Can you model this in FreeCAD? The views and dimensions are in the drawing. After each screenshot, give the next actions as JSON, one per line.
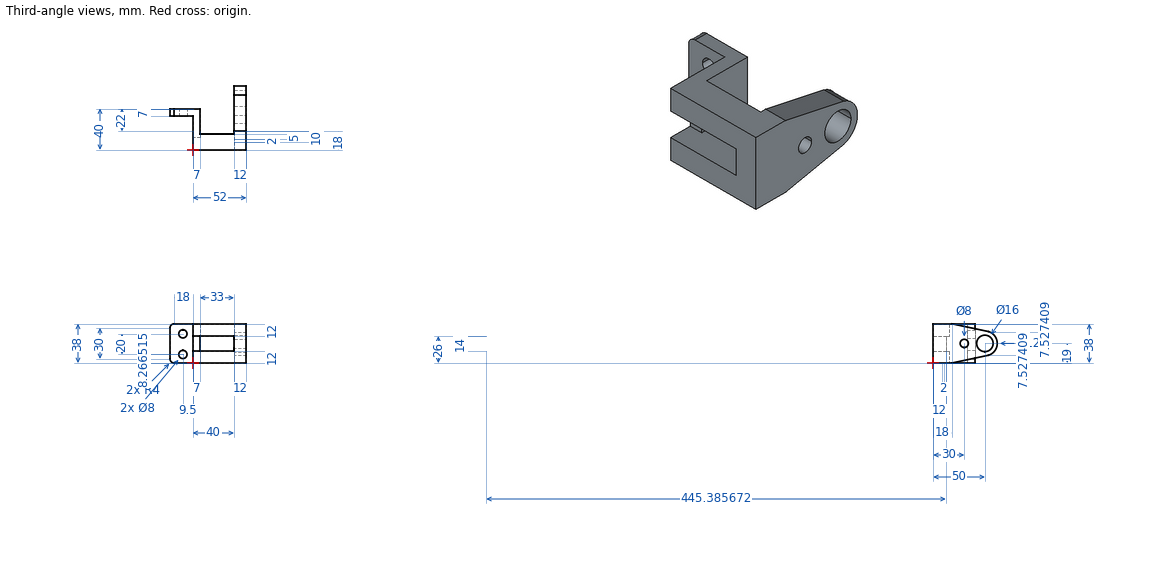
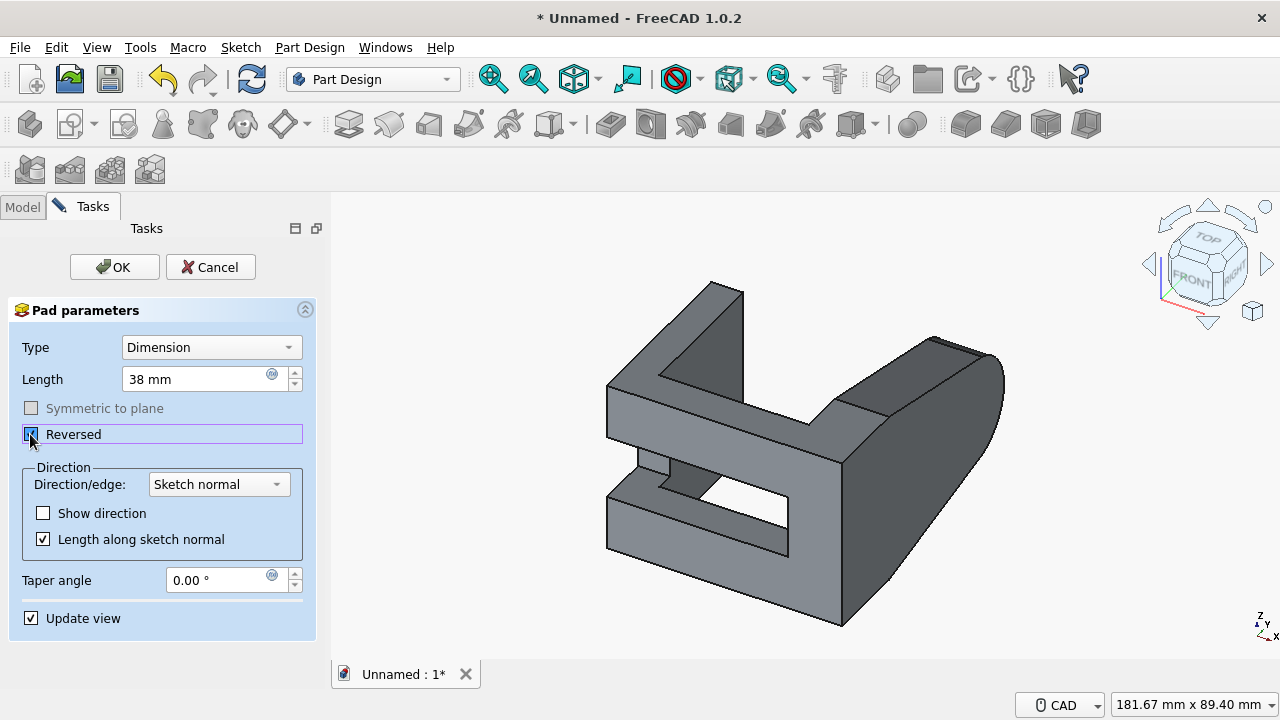
{"action": "left_click", "coordinate": [115, 267]}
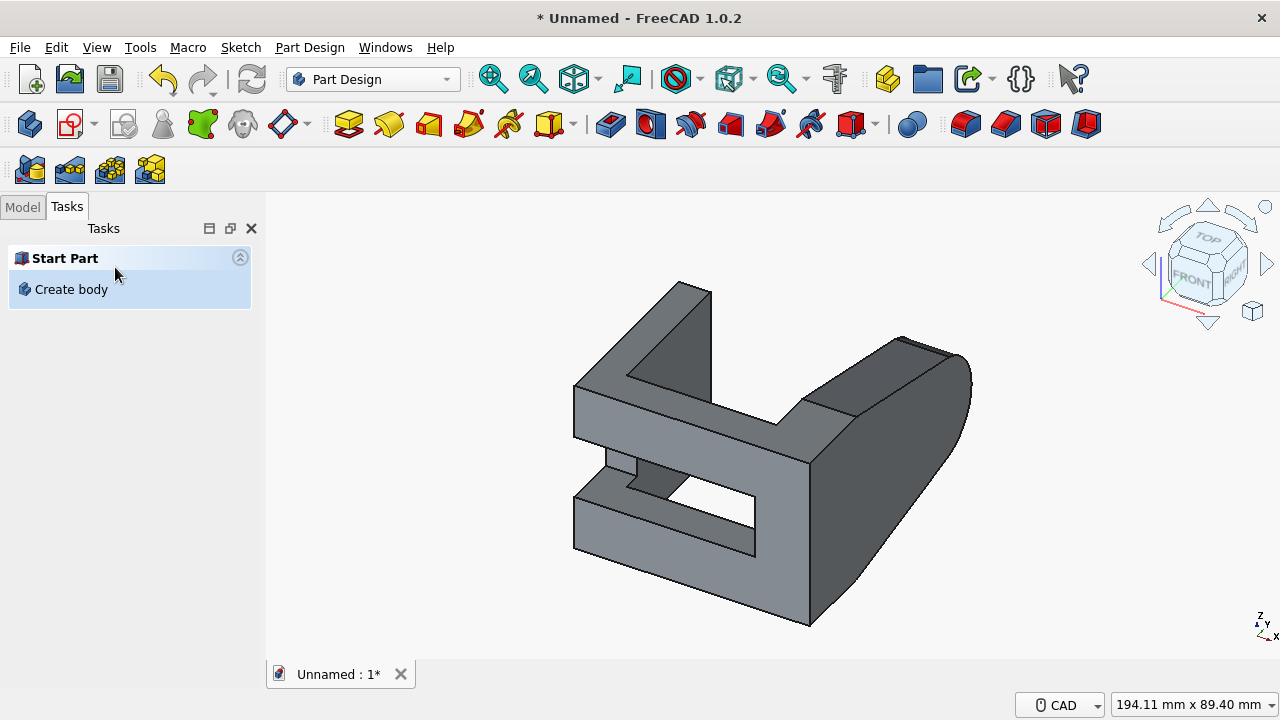
{"action": "key", "text": "4"}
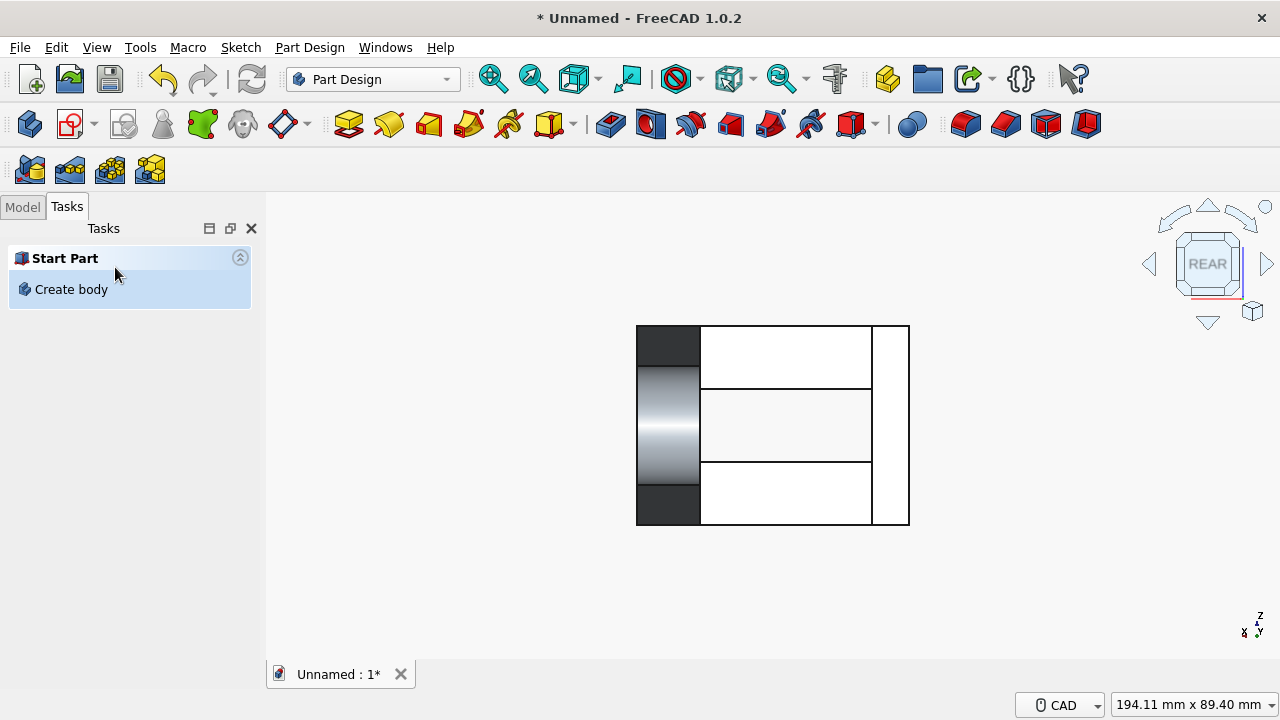
{"action": "left_click", "coordinate": [494, 80]}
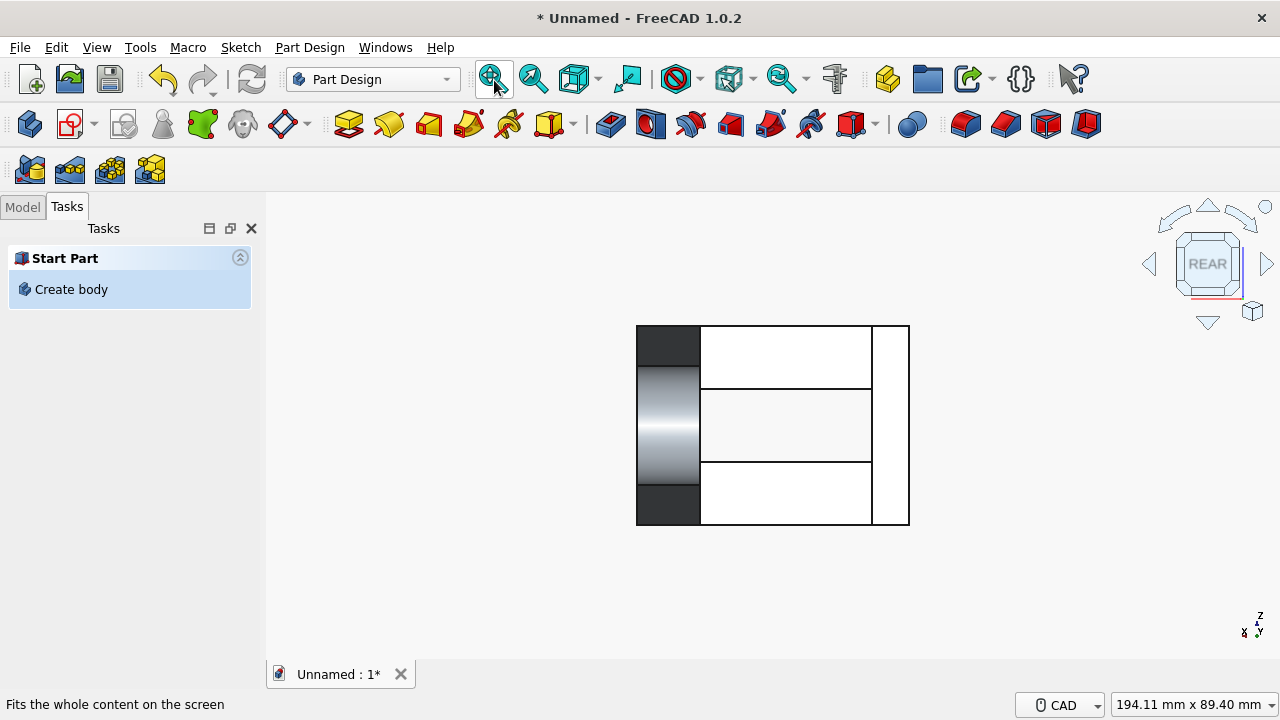
{"action": "left_click", "coordinate": [891, 368]}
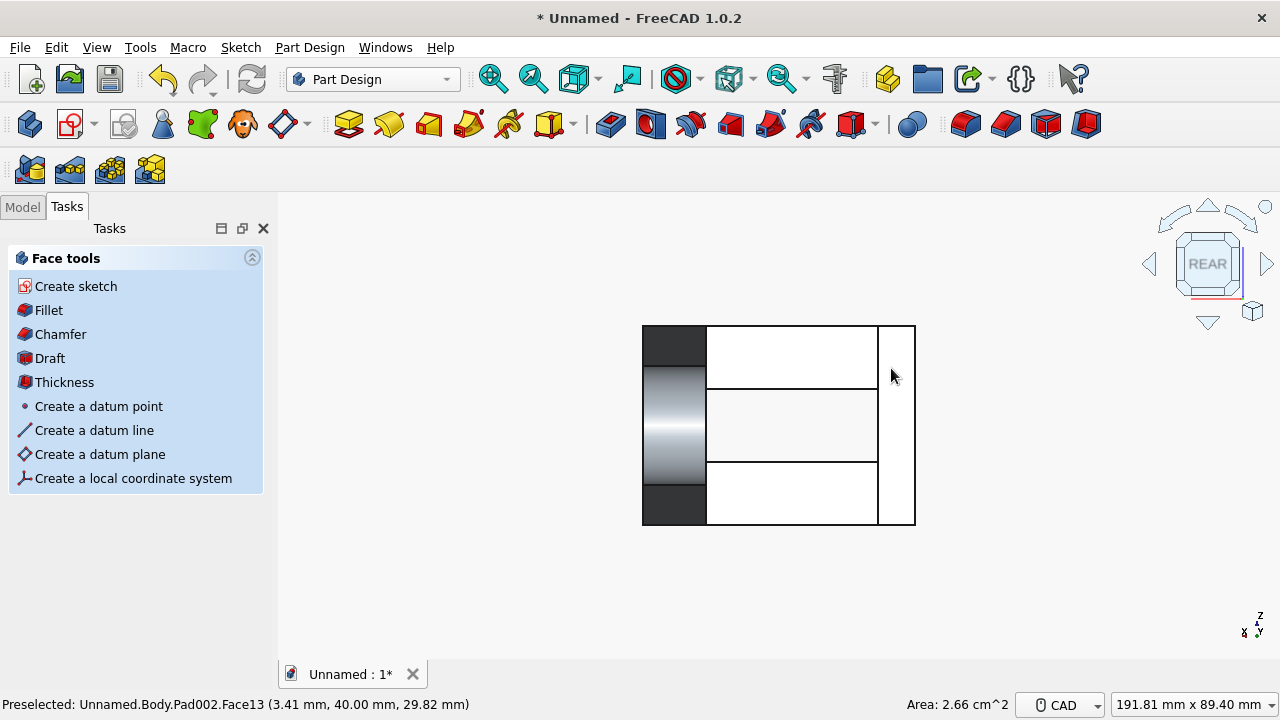
{"action": "left_click", "coordinate": [70, 124]}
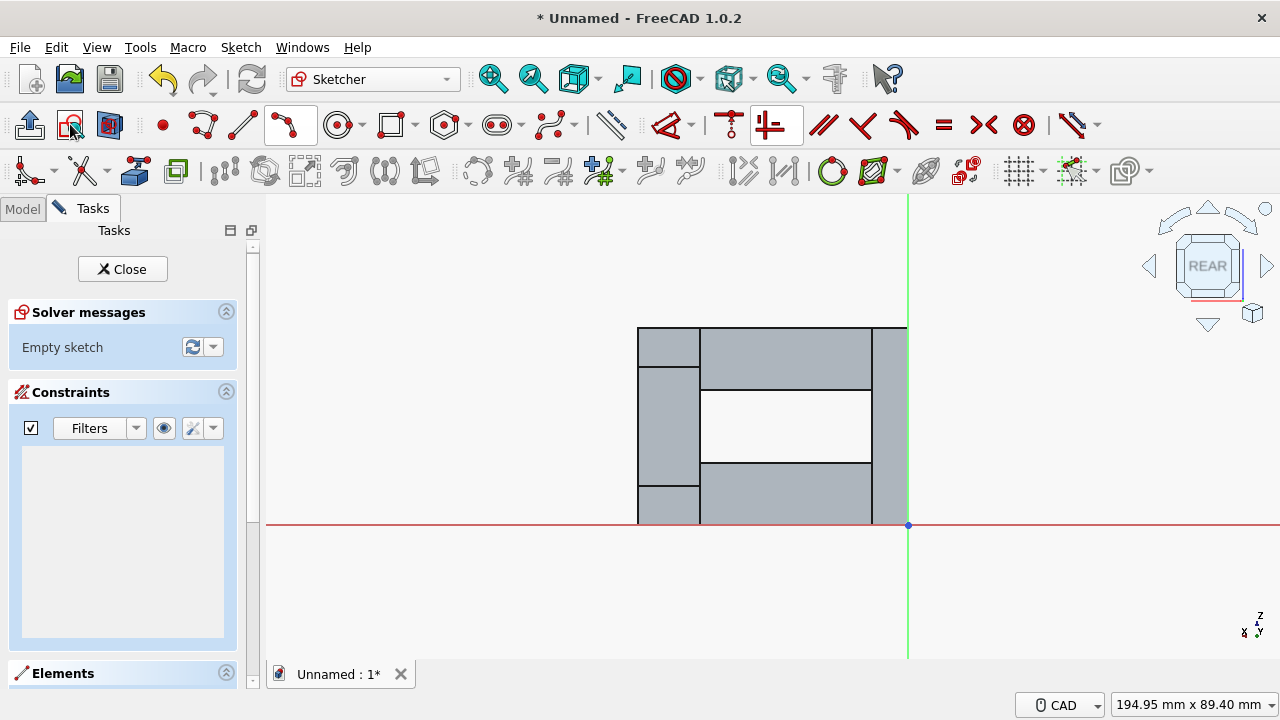
{"action": "left_click", "coordinate": [110, 126]}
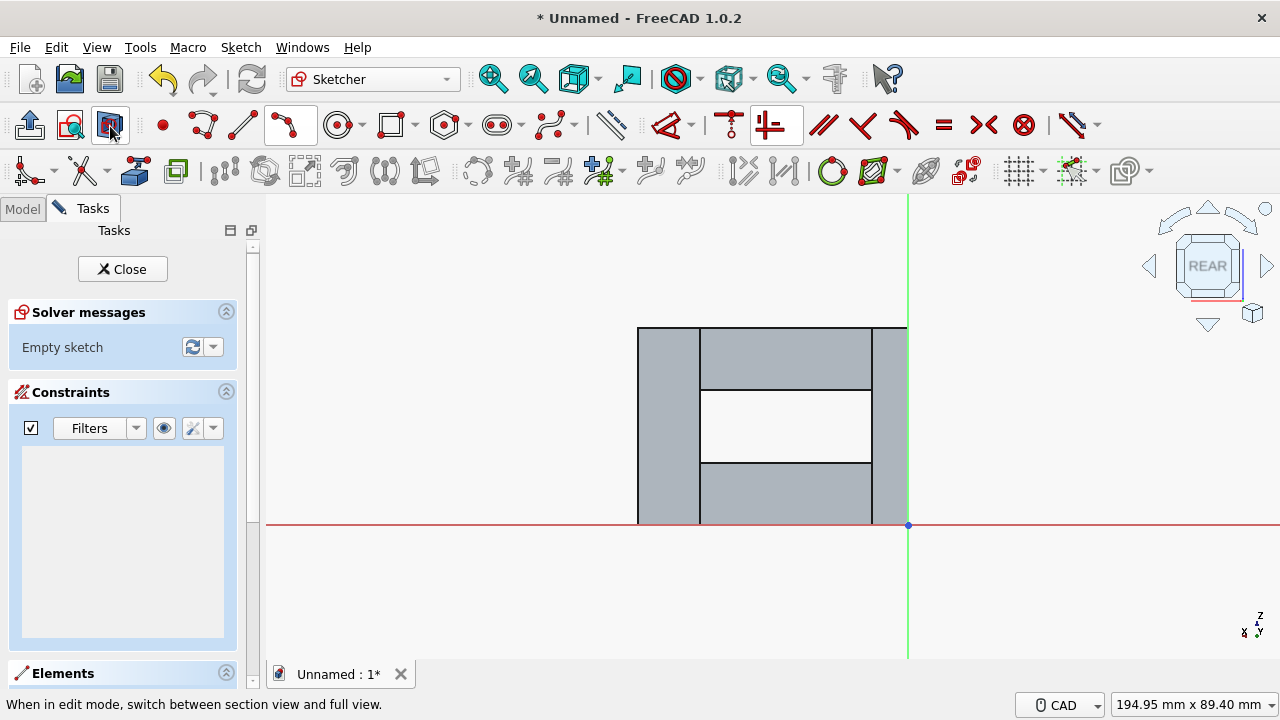
{"action": "scroll", "coordinate": [1115, 427], "scroll_direction": "up", "scroll_amount": 2}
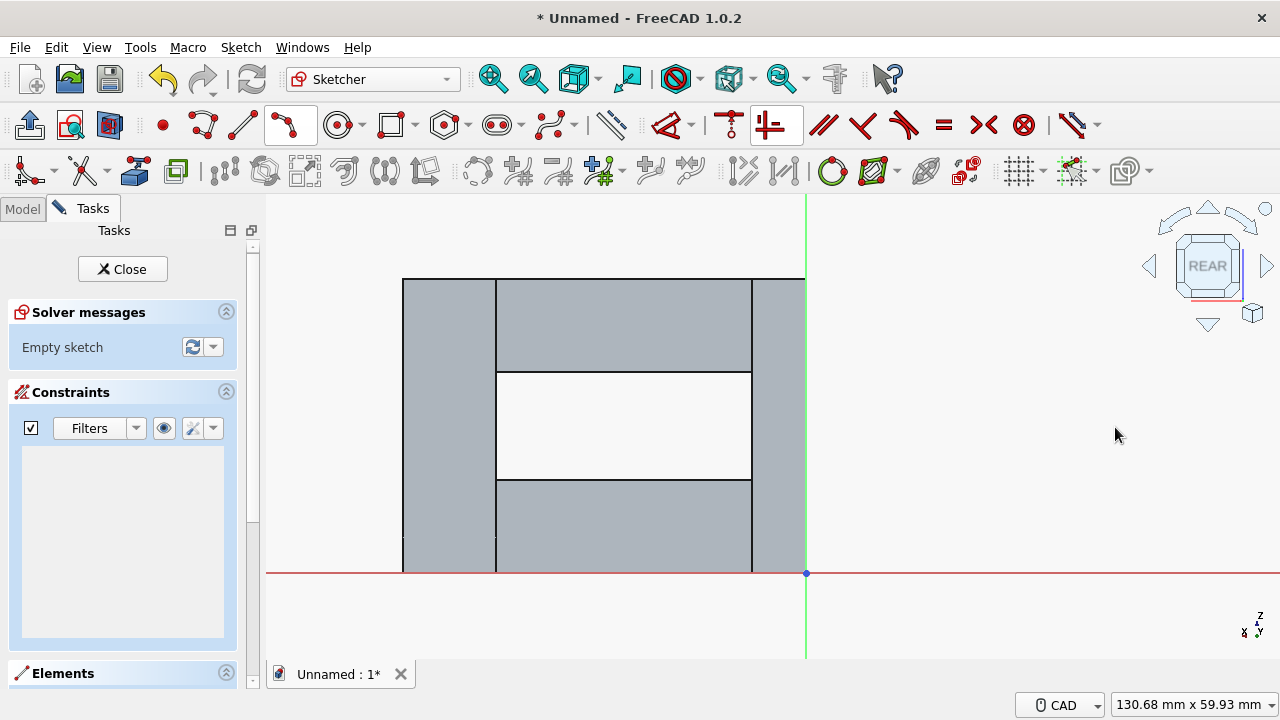
{"action": "left_click", "coordinate": [244, 126]}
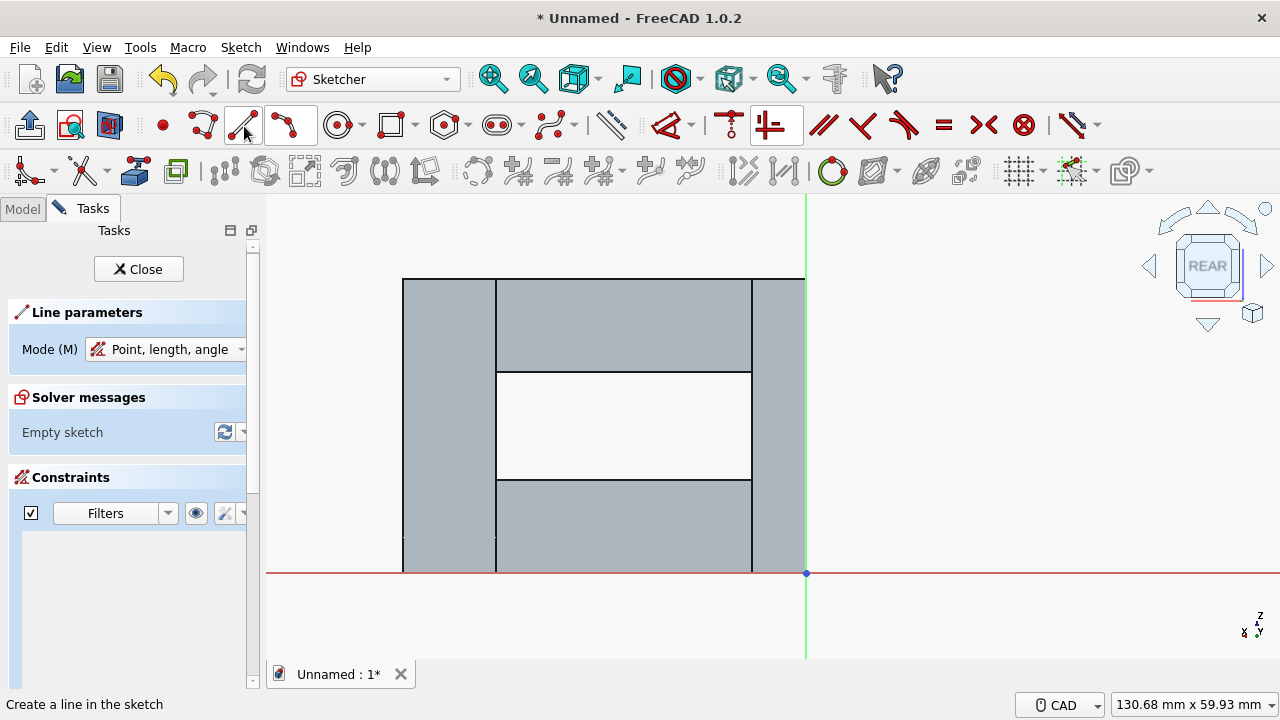
{"action": "left_click", "coordinate": [977, 542]}
{"action": "left_click", "coordinate": [977, 310]}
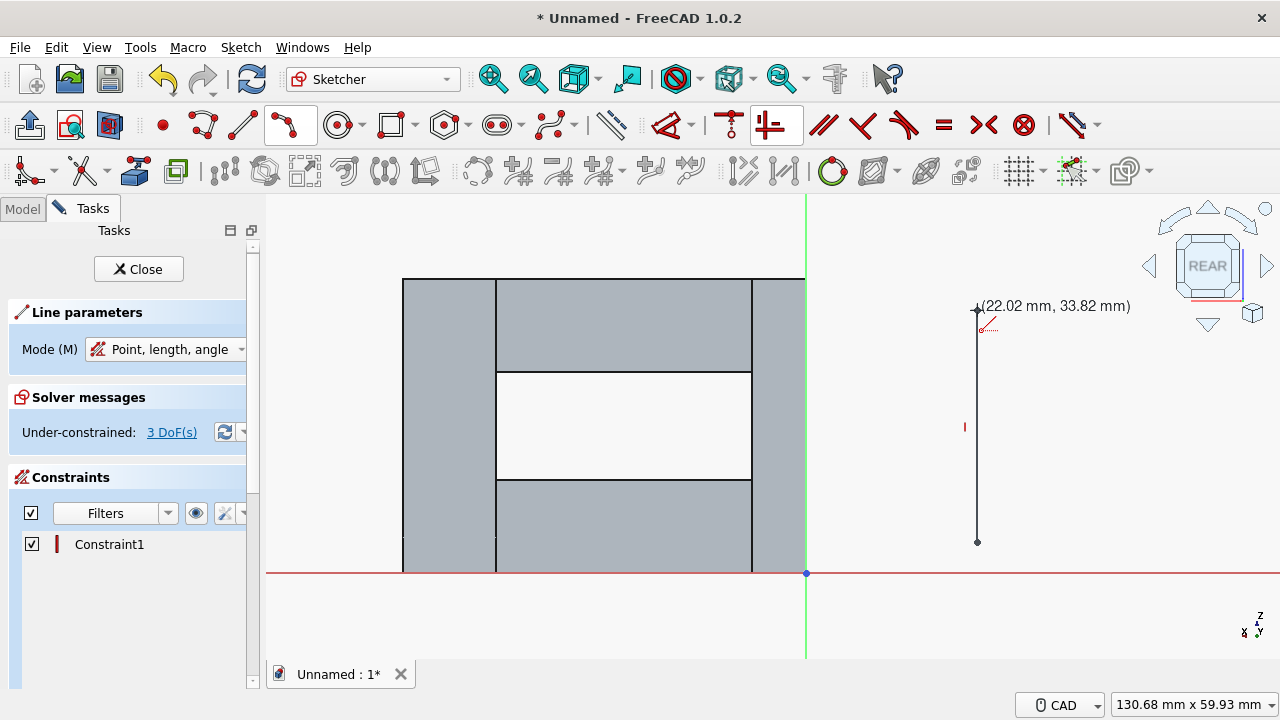
{"action": "left_click", "coordinate": [204, 126]}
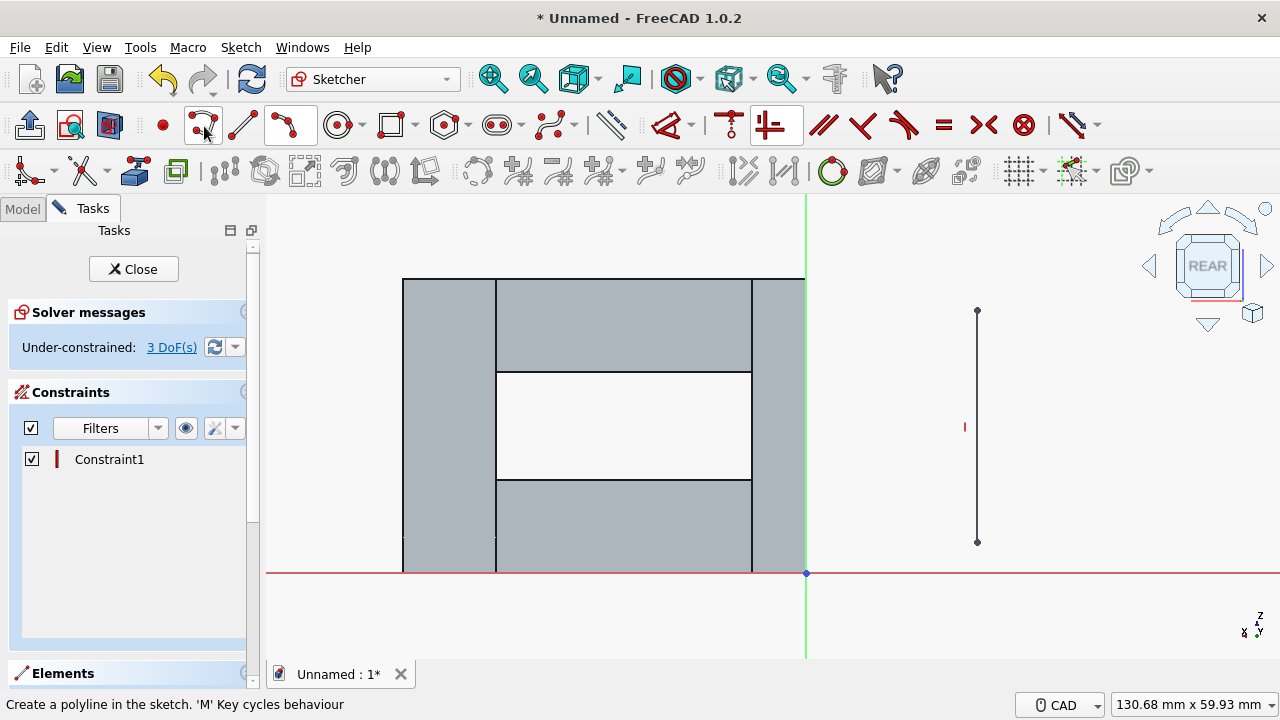
{"action": "left_click", "coordinate": [946, 279]}
{"action": "left_click", "coordinate": [806, 279]}
{"action": "left_click", "coordinate": [806, 573]}
{"action": "left_click", "coordinate": [946, 564]}
{"action": "right_click", "coordinate": [946, 564]}